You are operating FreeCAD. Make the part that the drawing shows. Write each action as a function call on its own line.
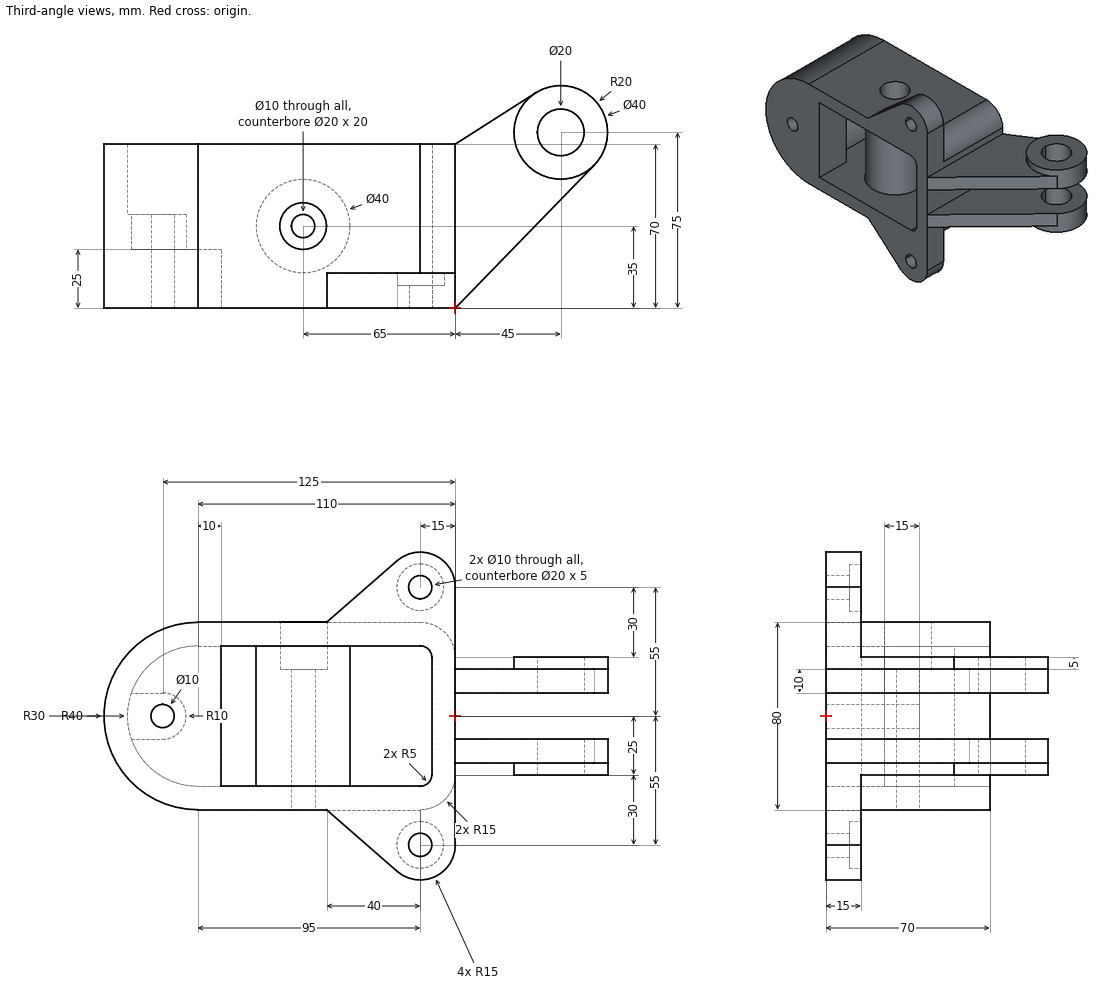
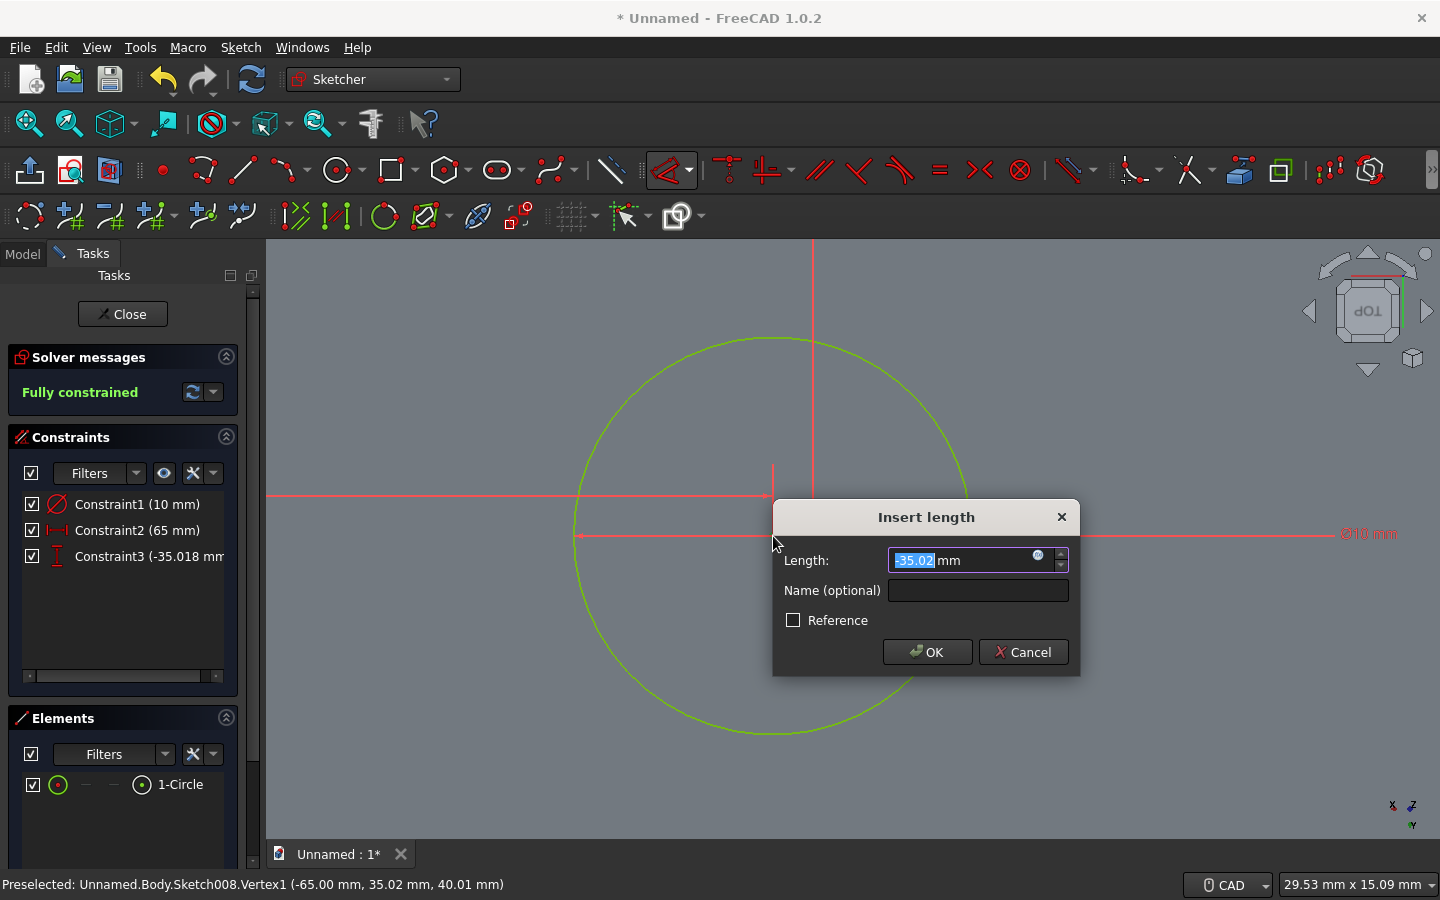
text(-35)
key(Return)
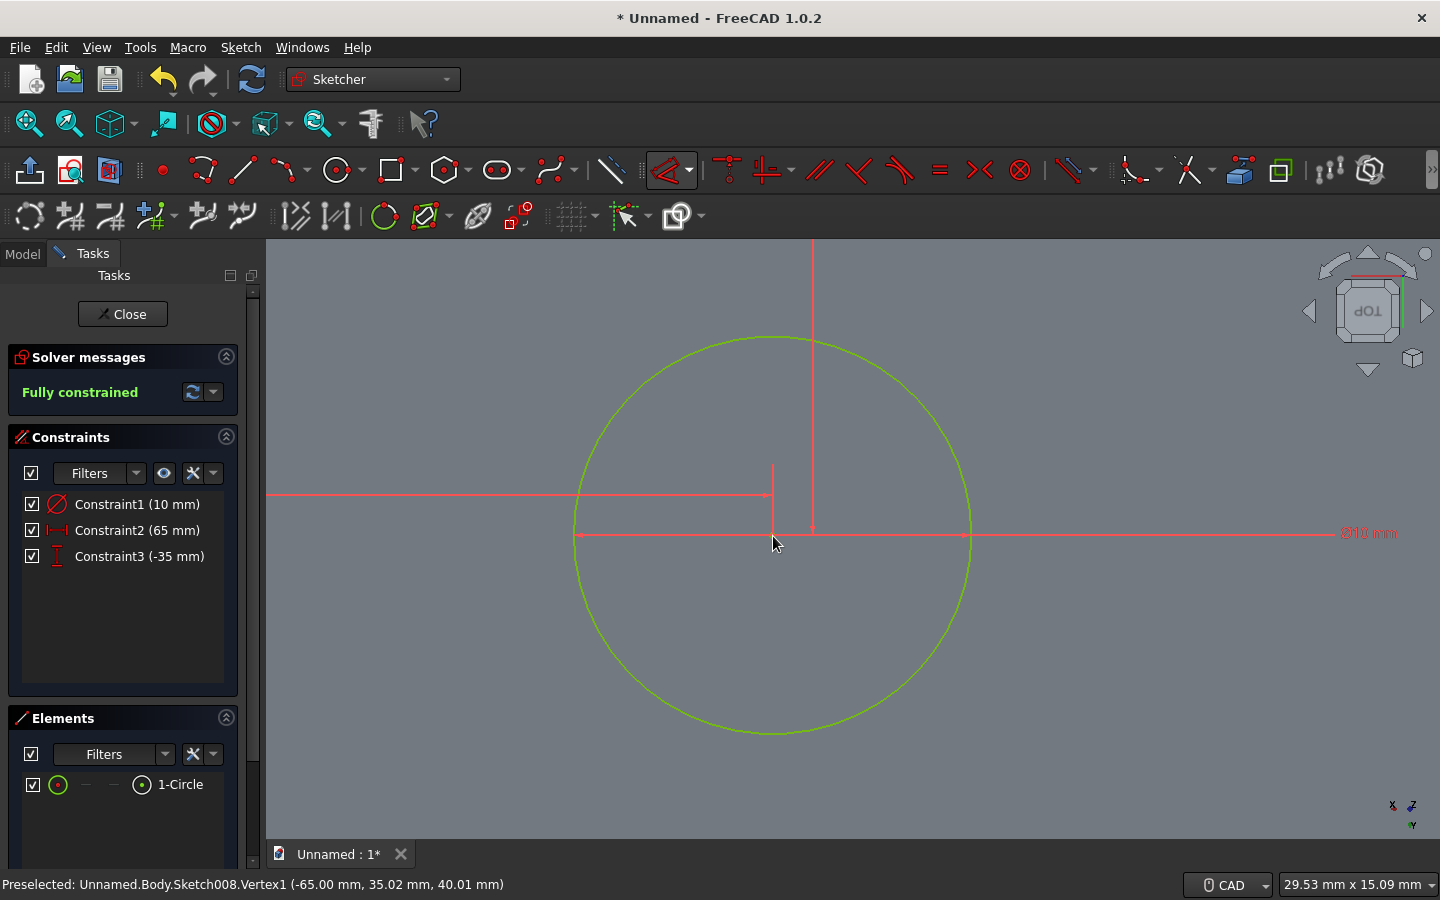
click(123, 314)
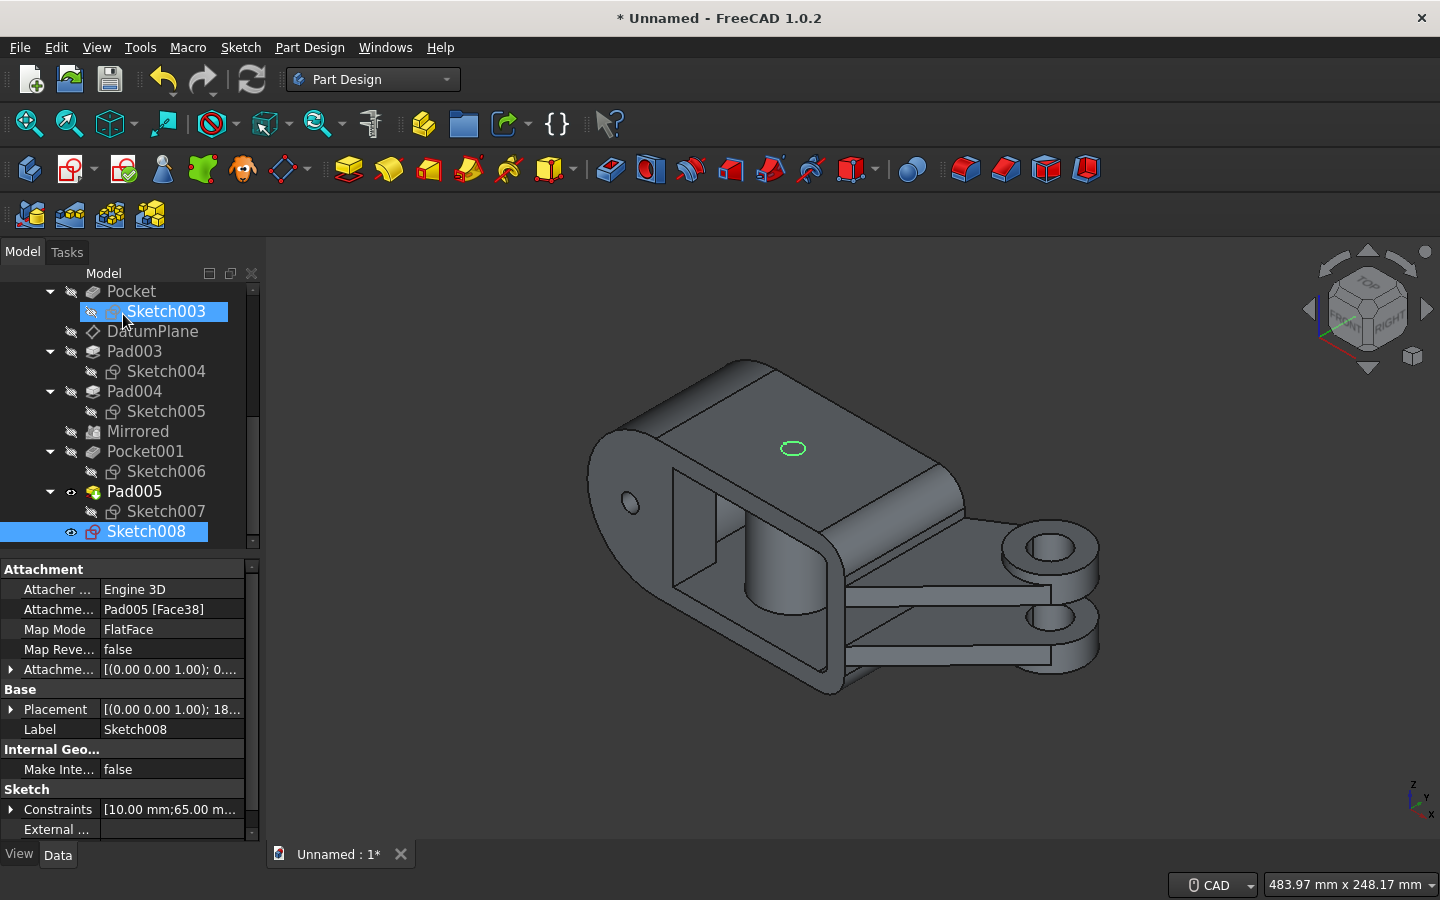
click(652, 170)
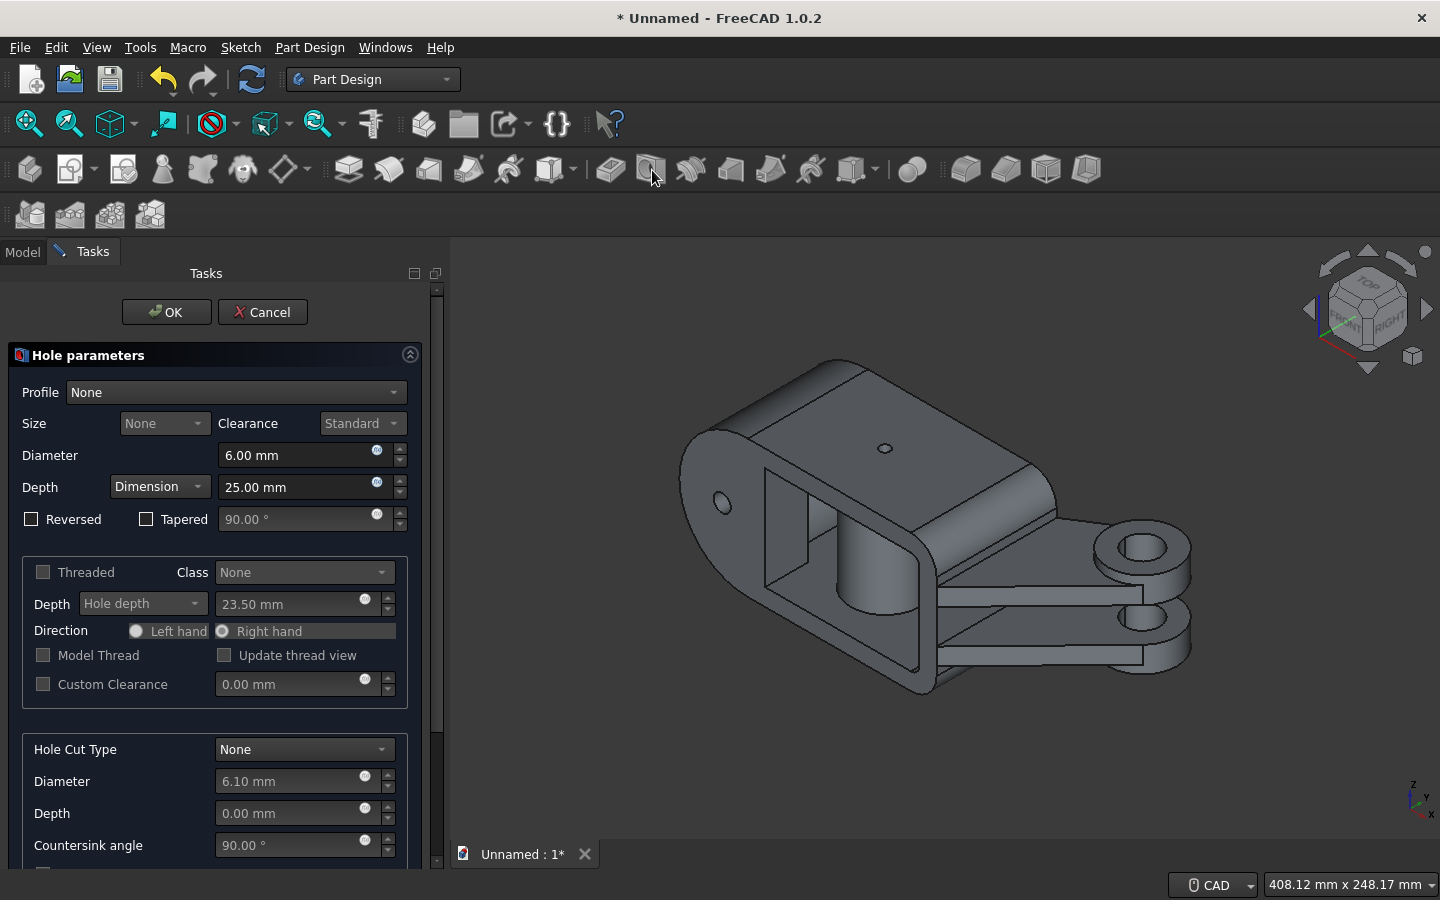
triple_click(305, 455)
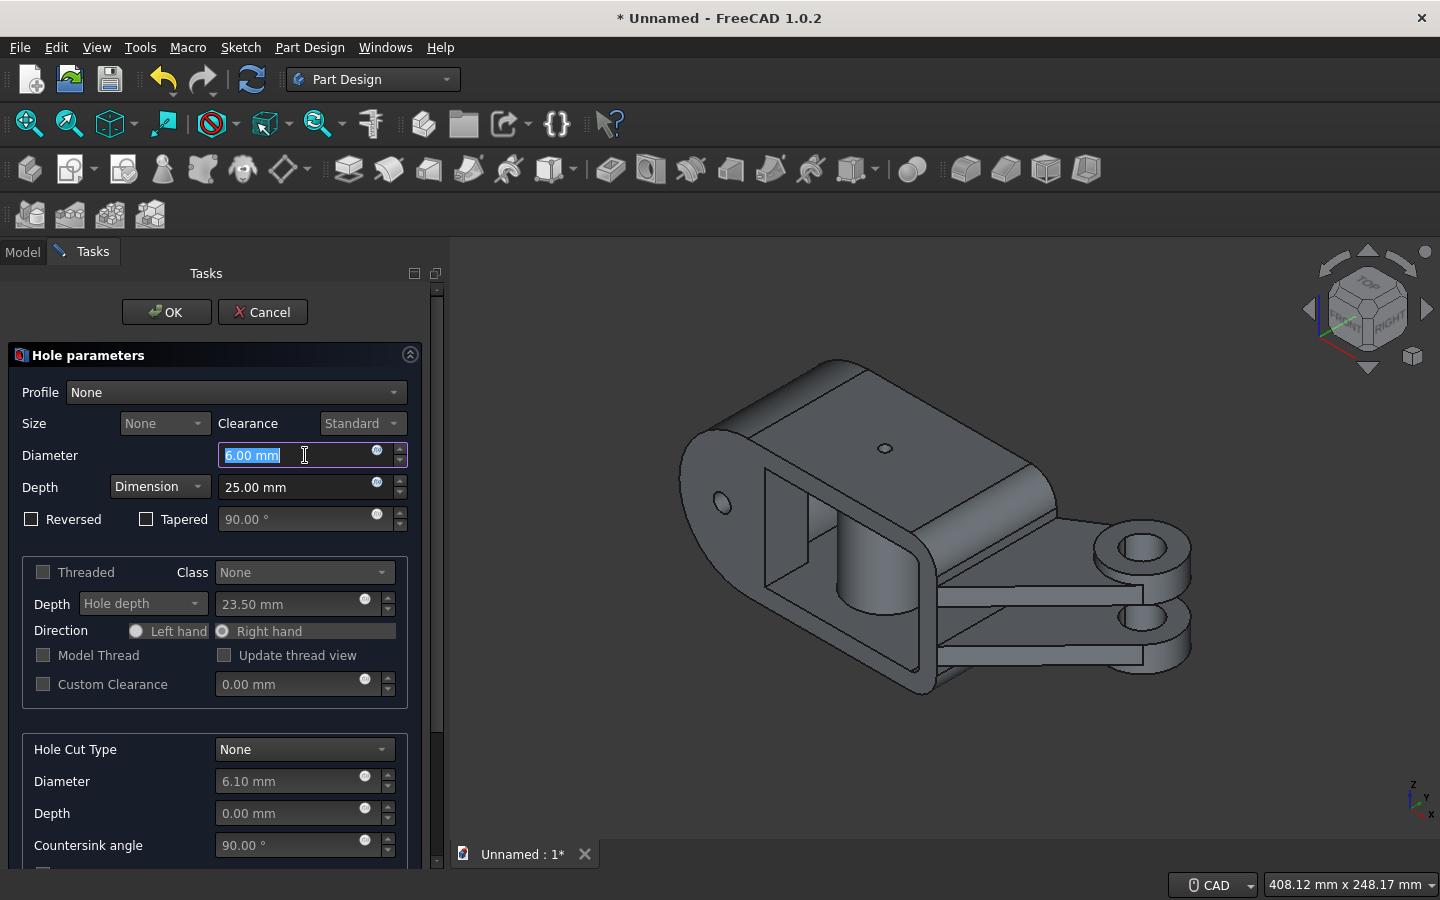
text(10)
key(Tab)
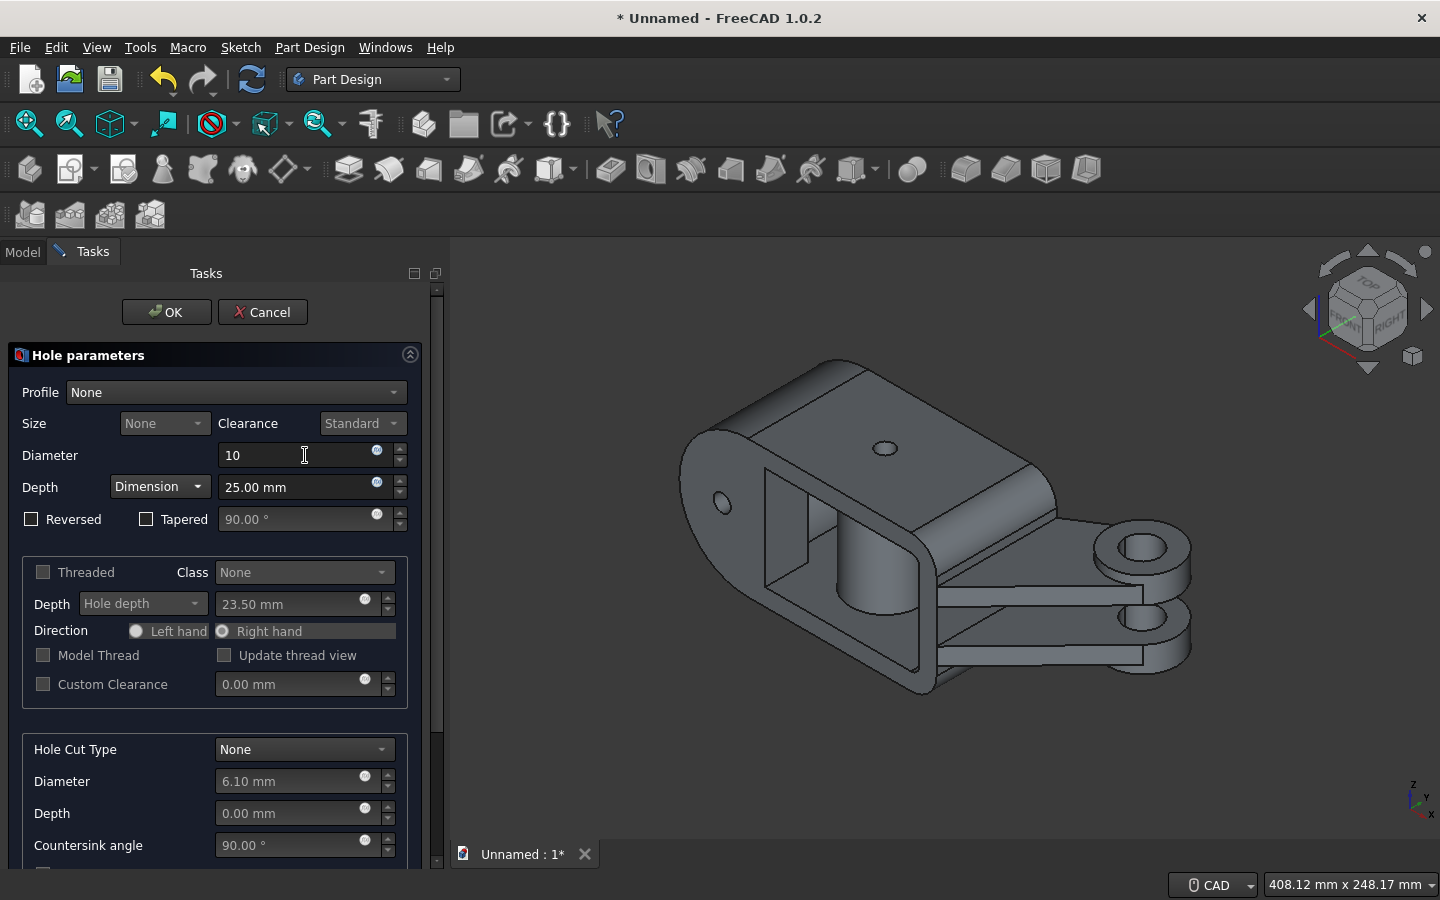
click(161, 486)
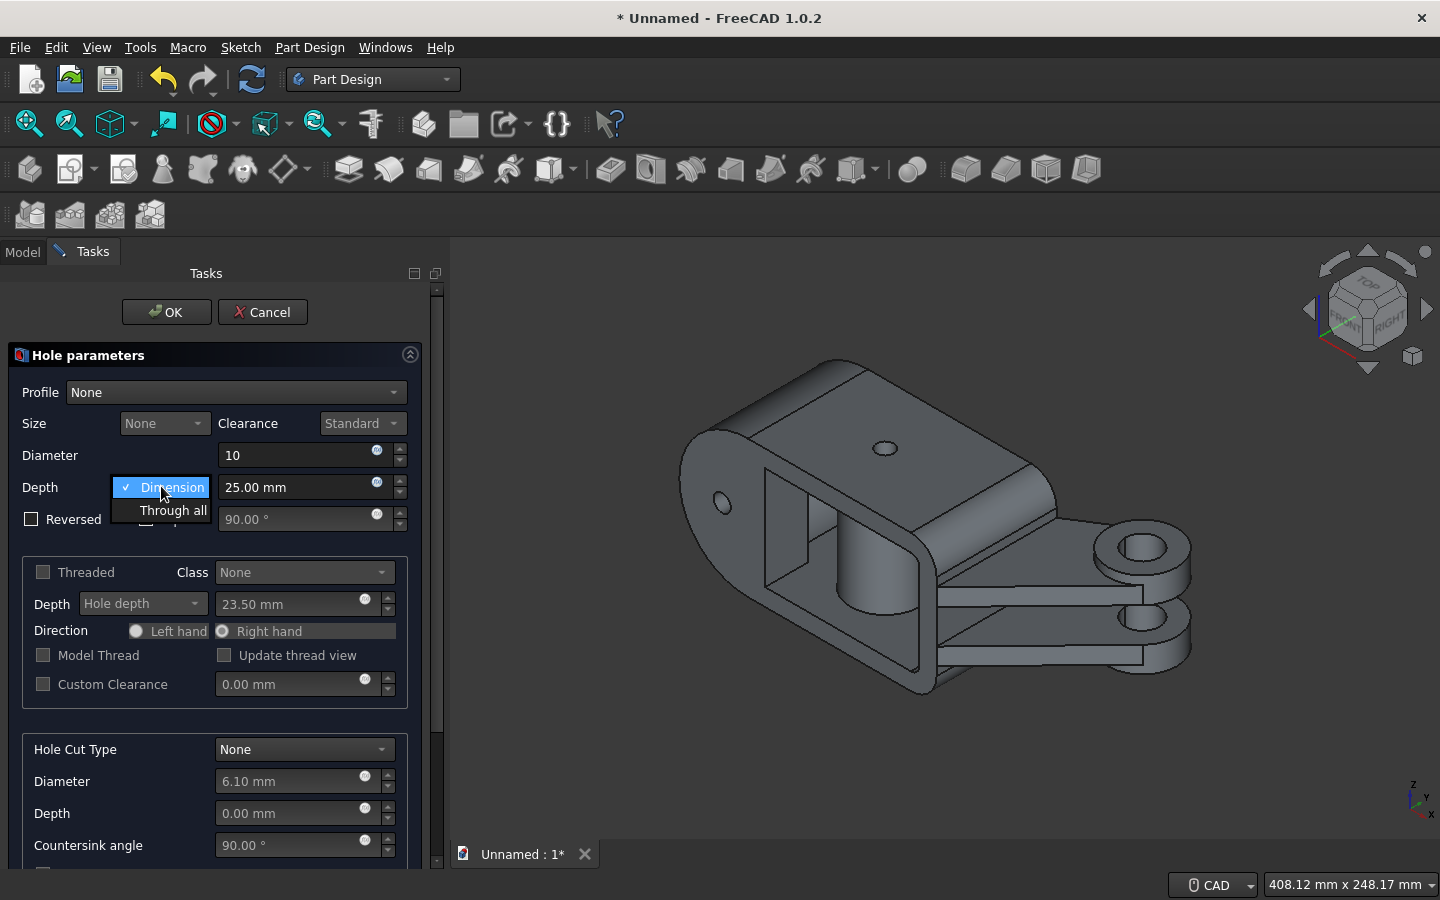
click(160, 510)